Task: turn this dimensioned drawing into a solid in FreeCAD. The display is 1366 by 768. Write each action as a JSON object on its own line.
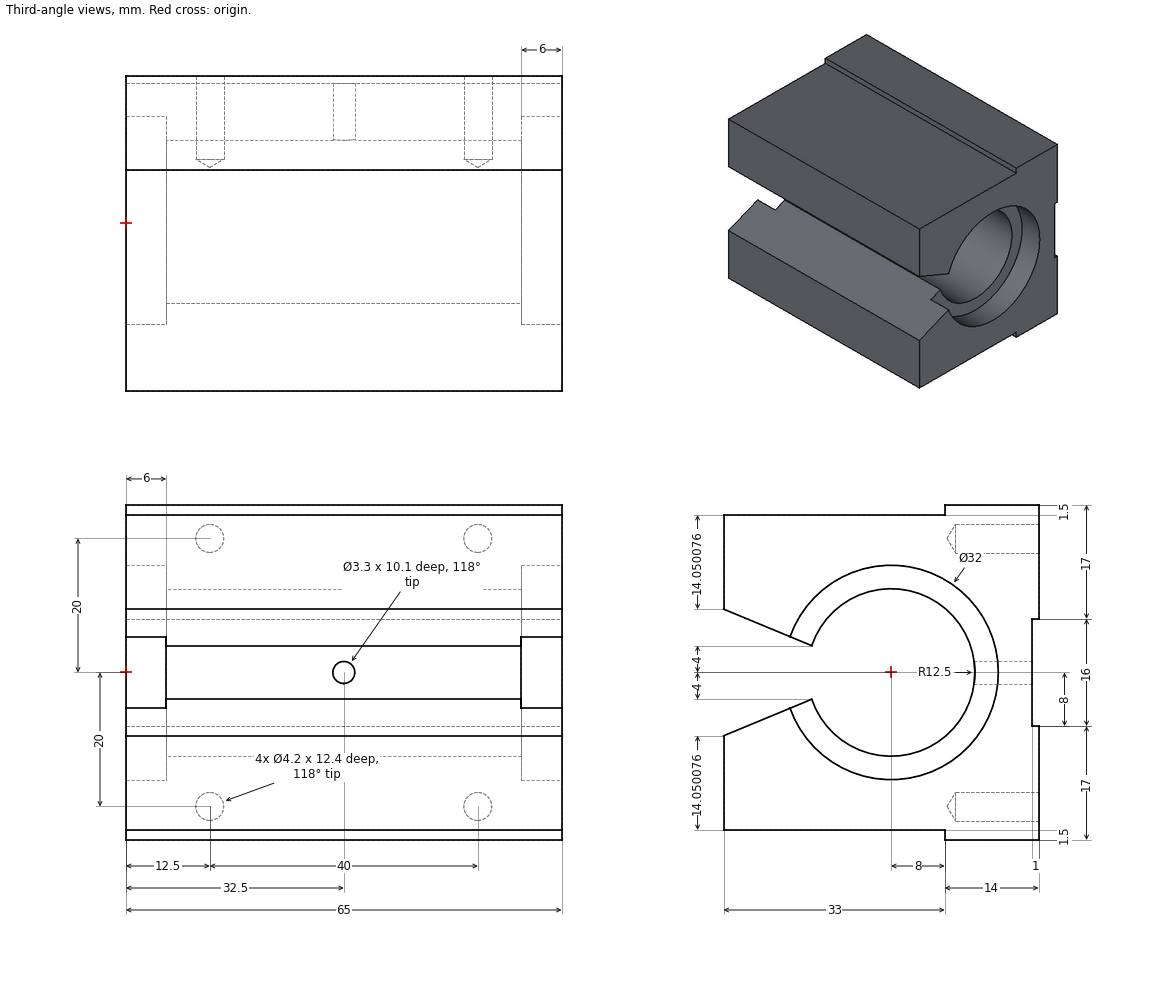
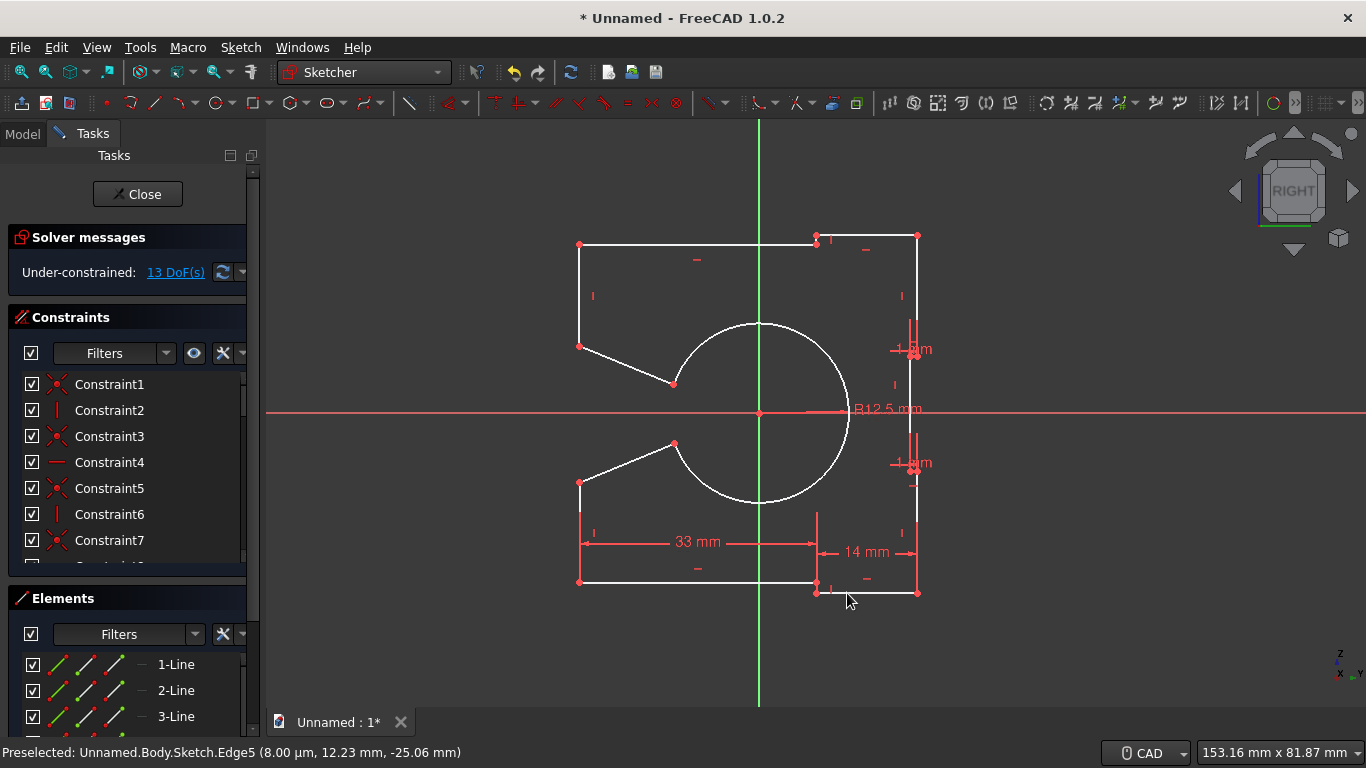
{"action": "left_click", "coordinate": [917, 556]}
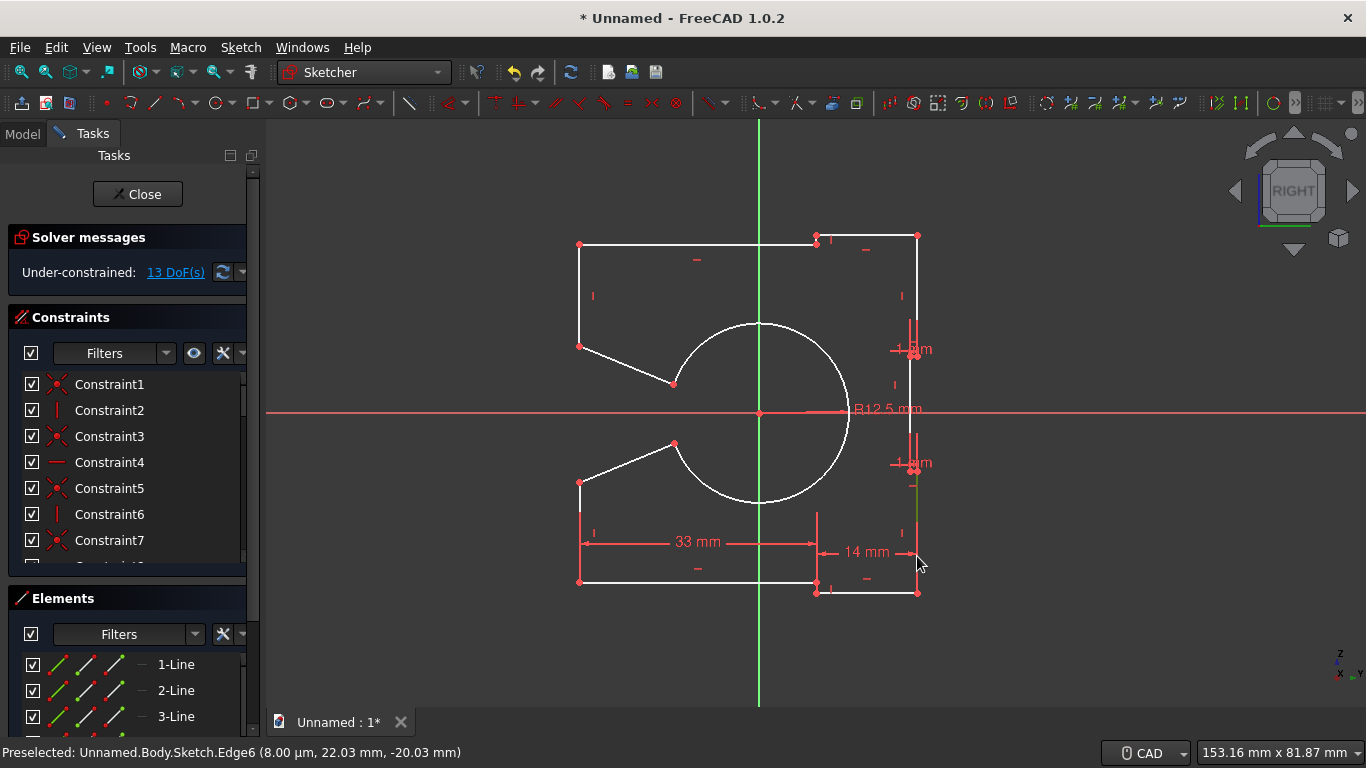
{"action": "key", "text": "i"}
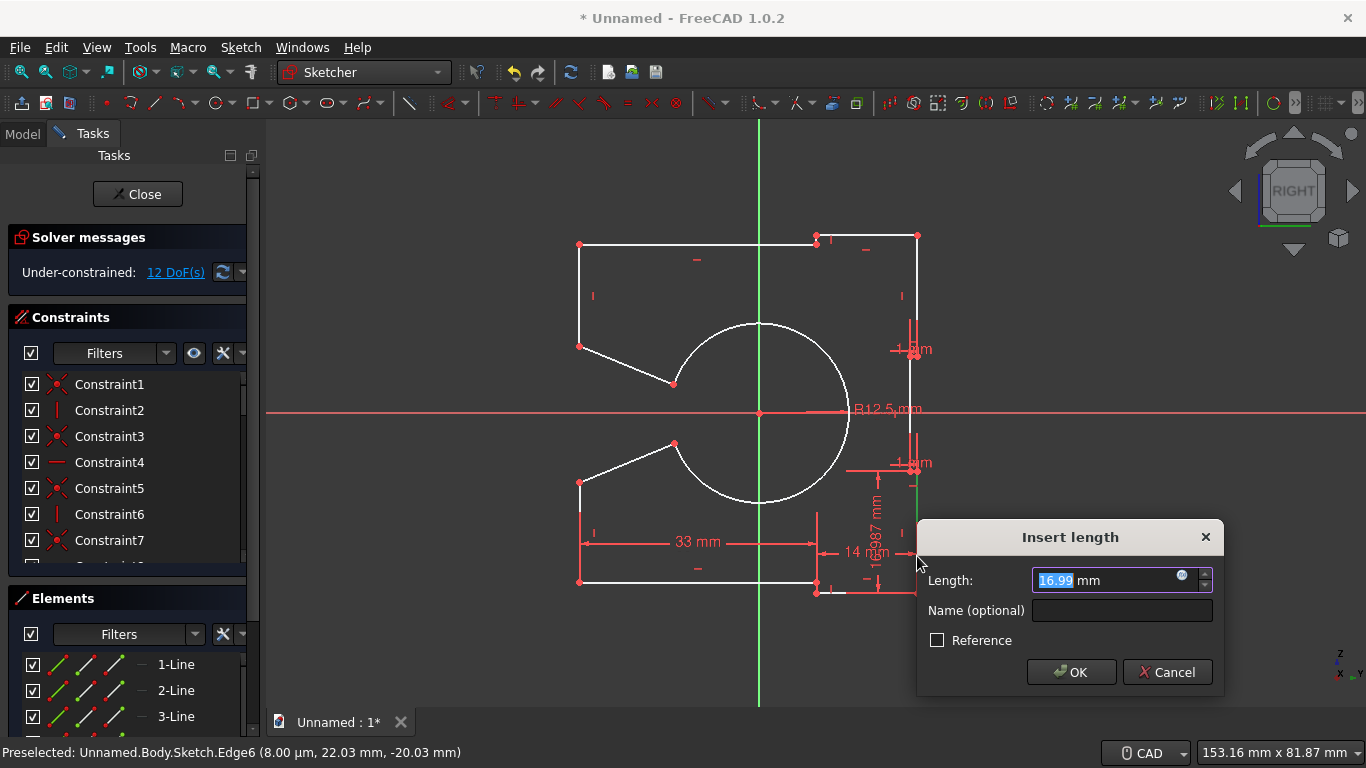
{"action": "type", "text": "17"}
{"action": "key", "text": "Return"}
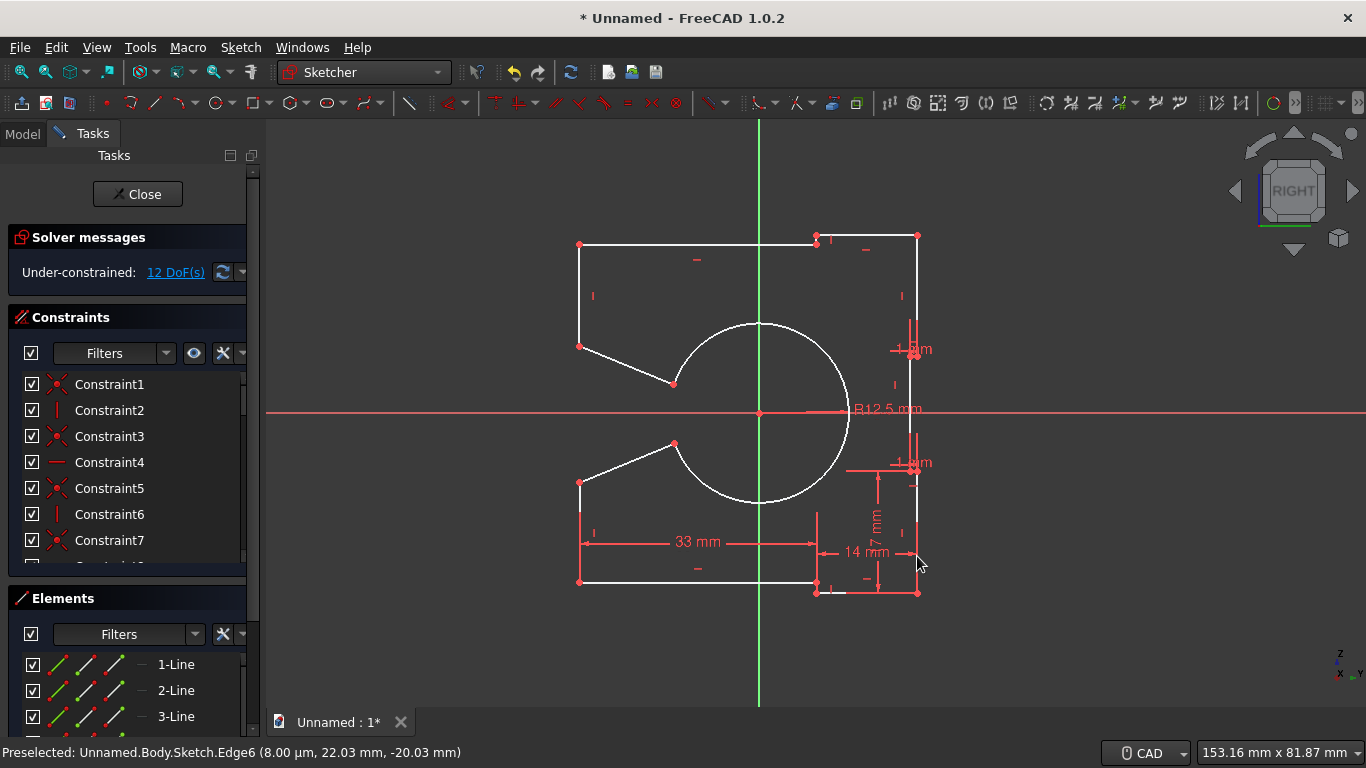
{"action": "left_click", "coordinate": [910, 437]}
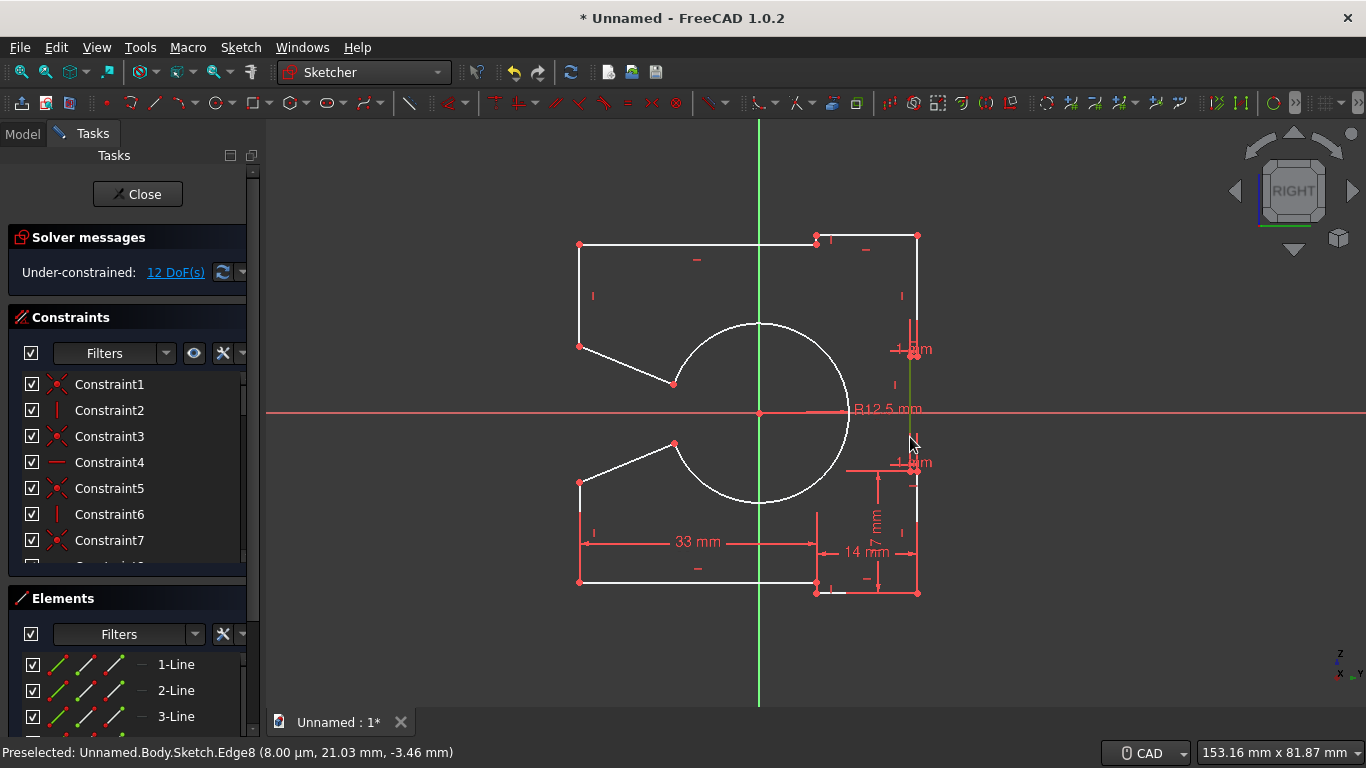
{"action": "key", "text": "i"}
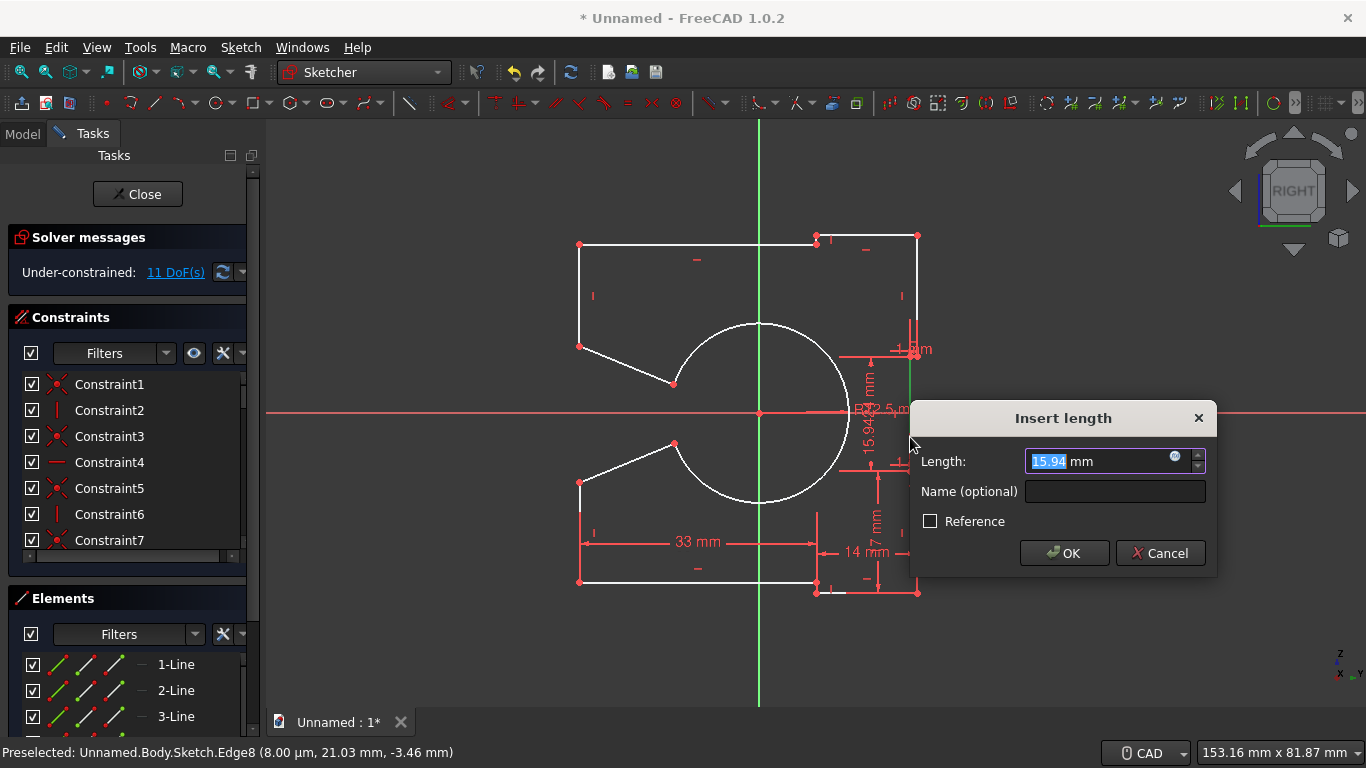
{"action": "type", "text": "16"}
{"action": "key", "text": "Return"}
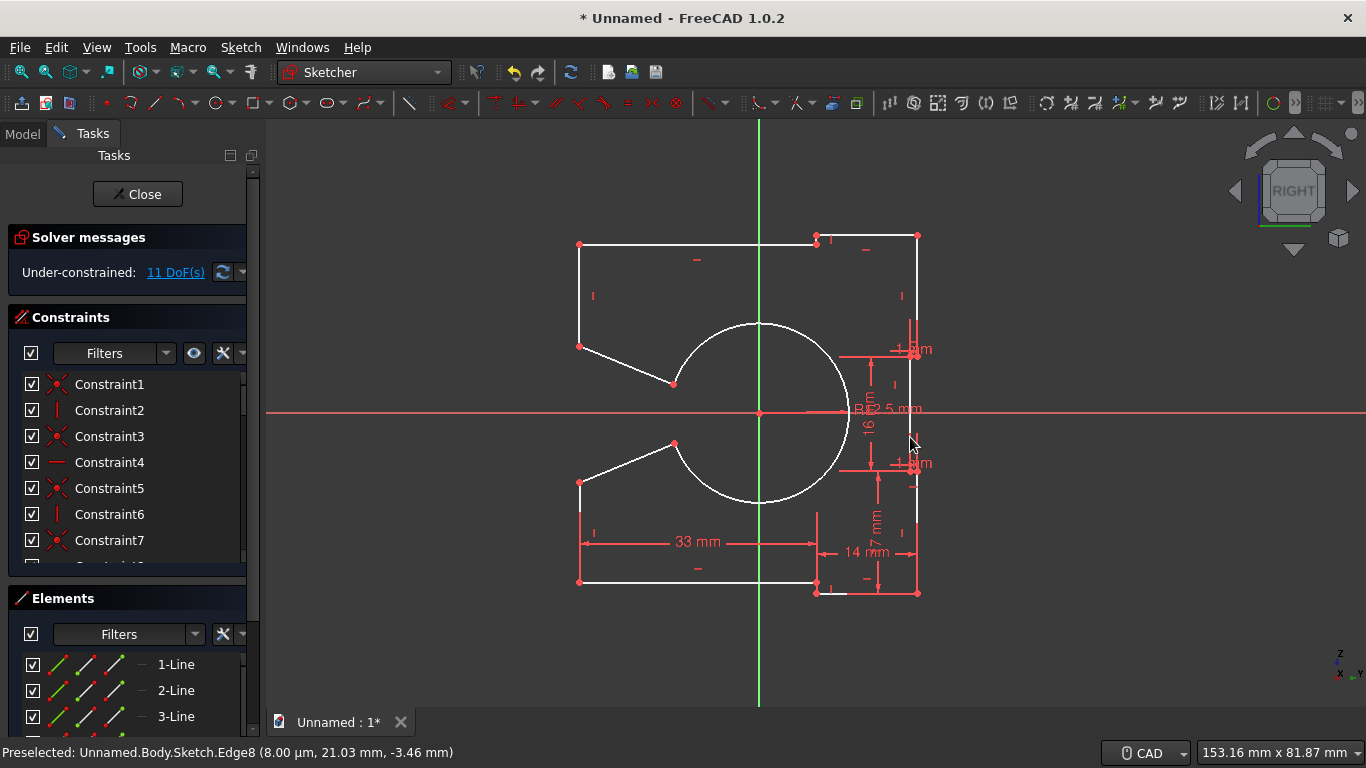
{"action": "left_click", "coordinate": [917, 320]}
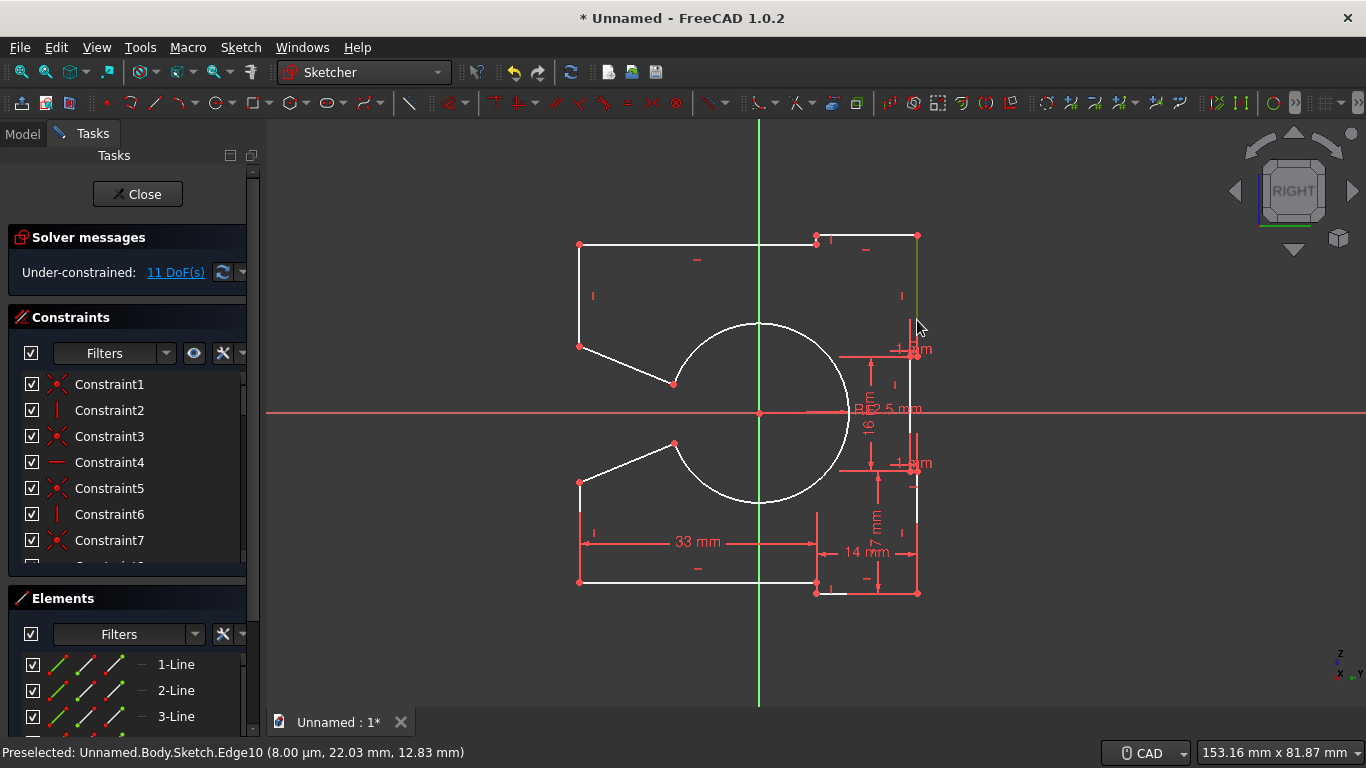
{"action": "key", "text": "i"}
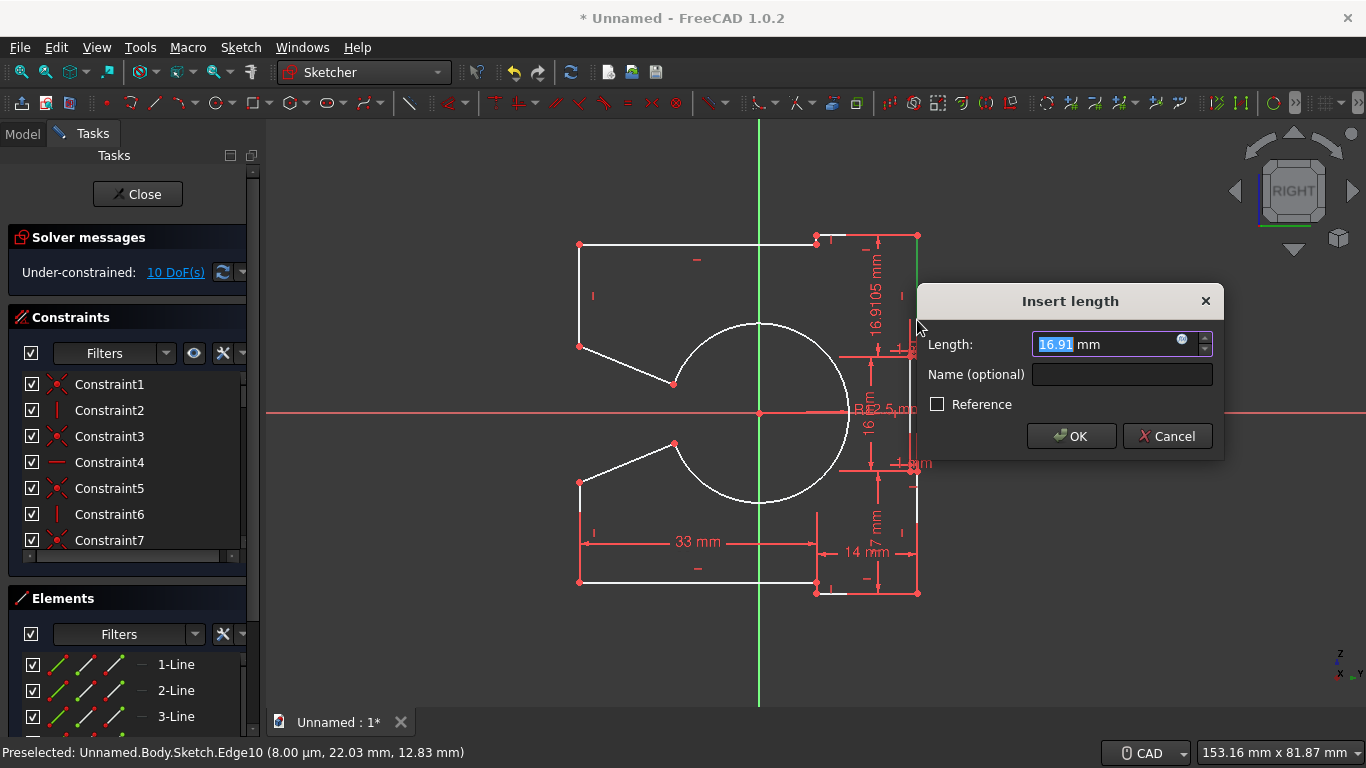
{"action": "type", "text": "17"}
{"action": "key", "text": "Return"}